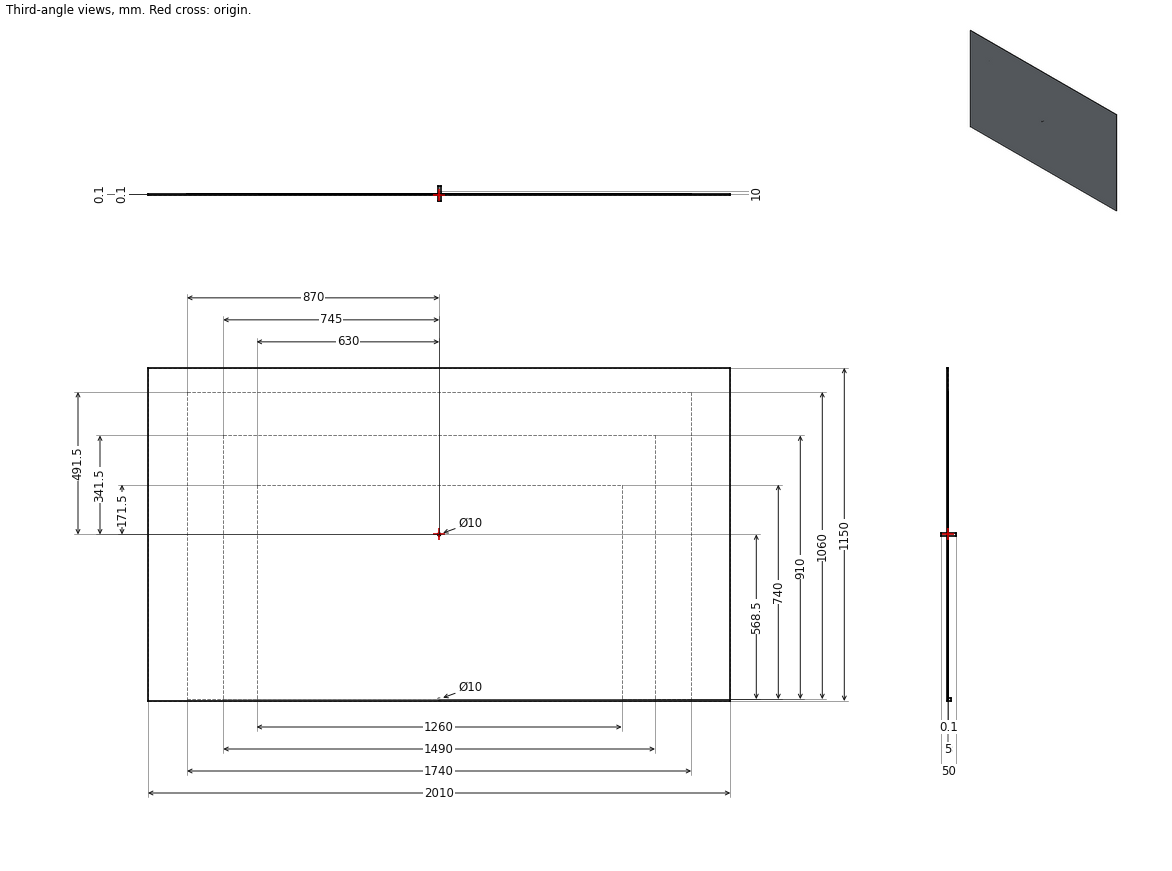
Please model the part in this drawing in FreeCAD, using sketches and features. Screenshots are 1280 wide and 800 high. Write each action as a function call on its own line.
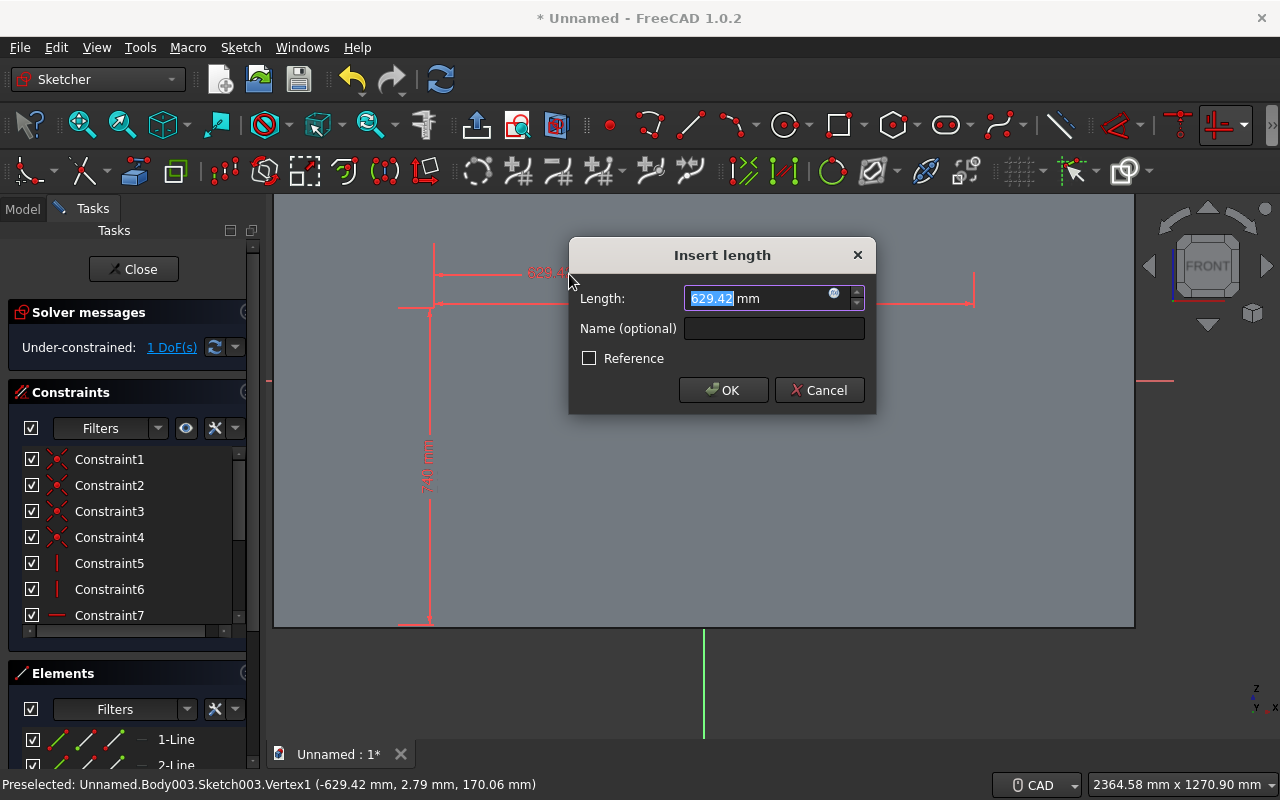
text(630)
key(Return)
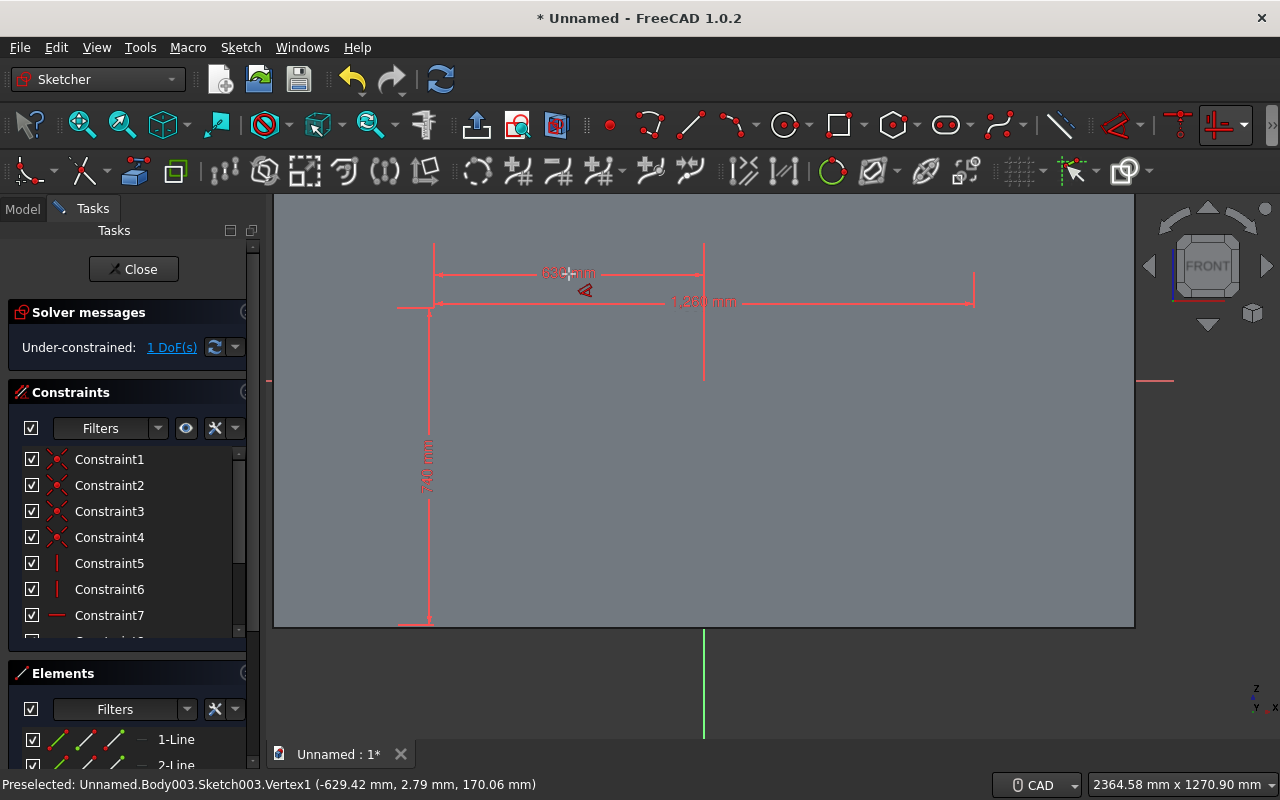
click(434, 308)
click(400, 344)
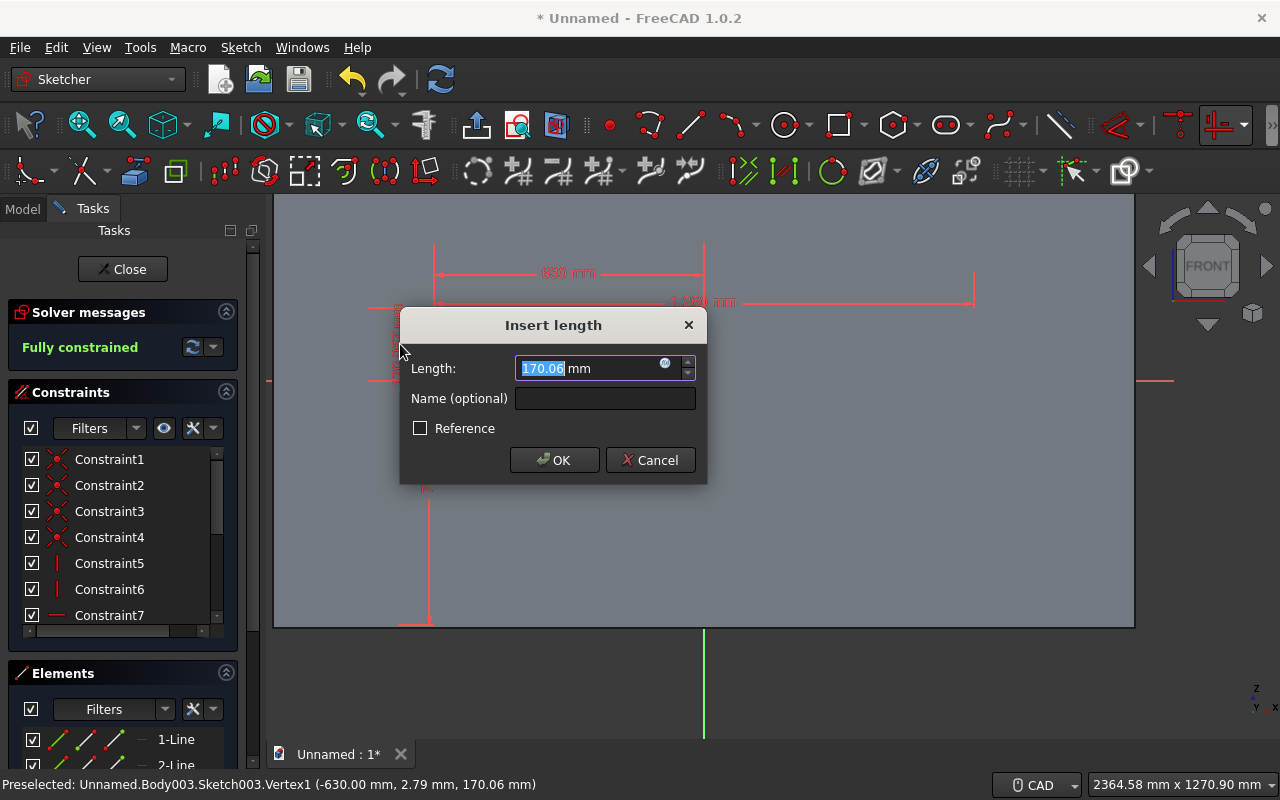
text(171.5)
key(Return)
key(Escape)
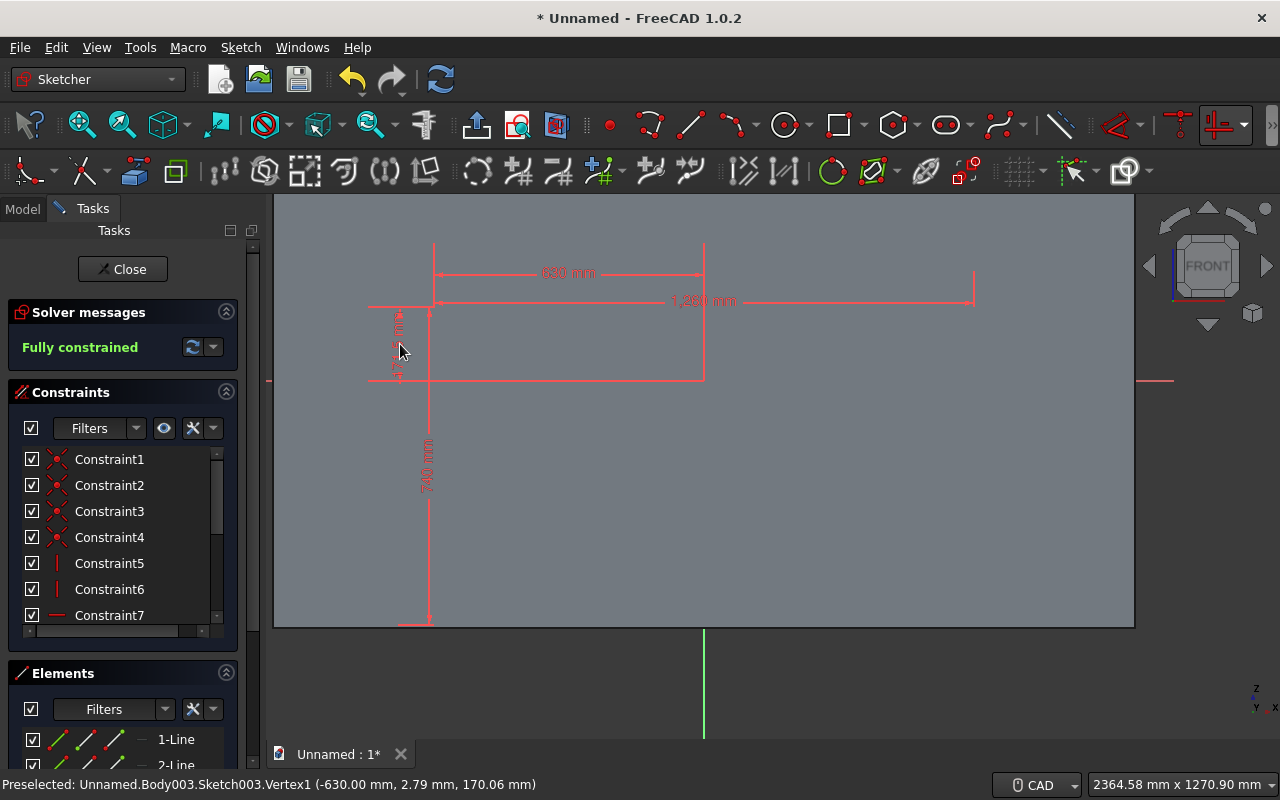
click(123, 269)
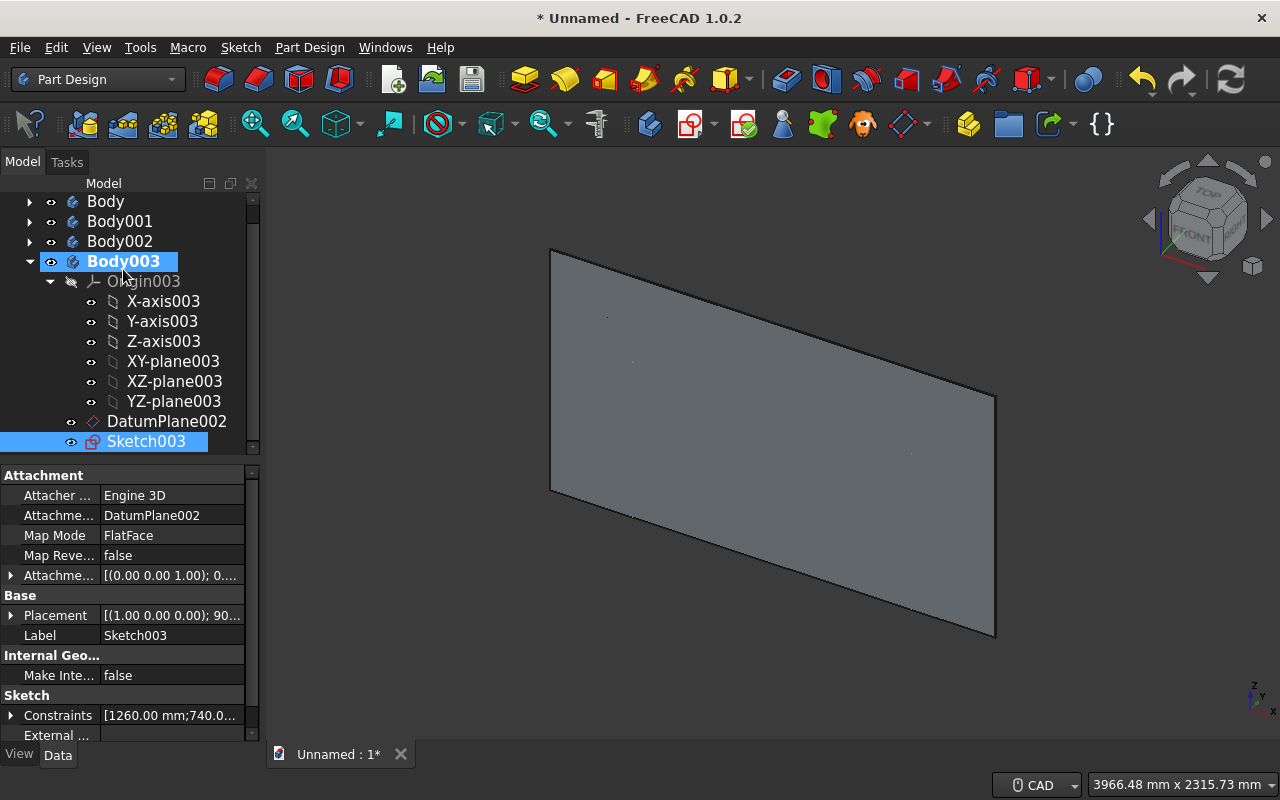
click(526, 80)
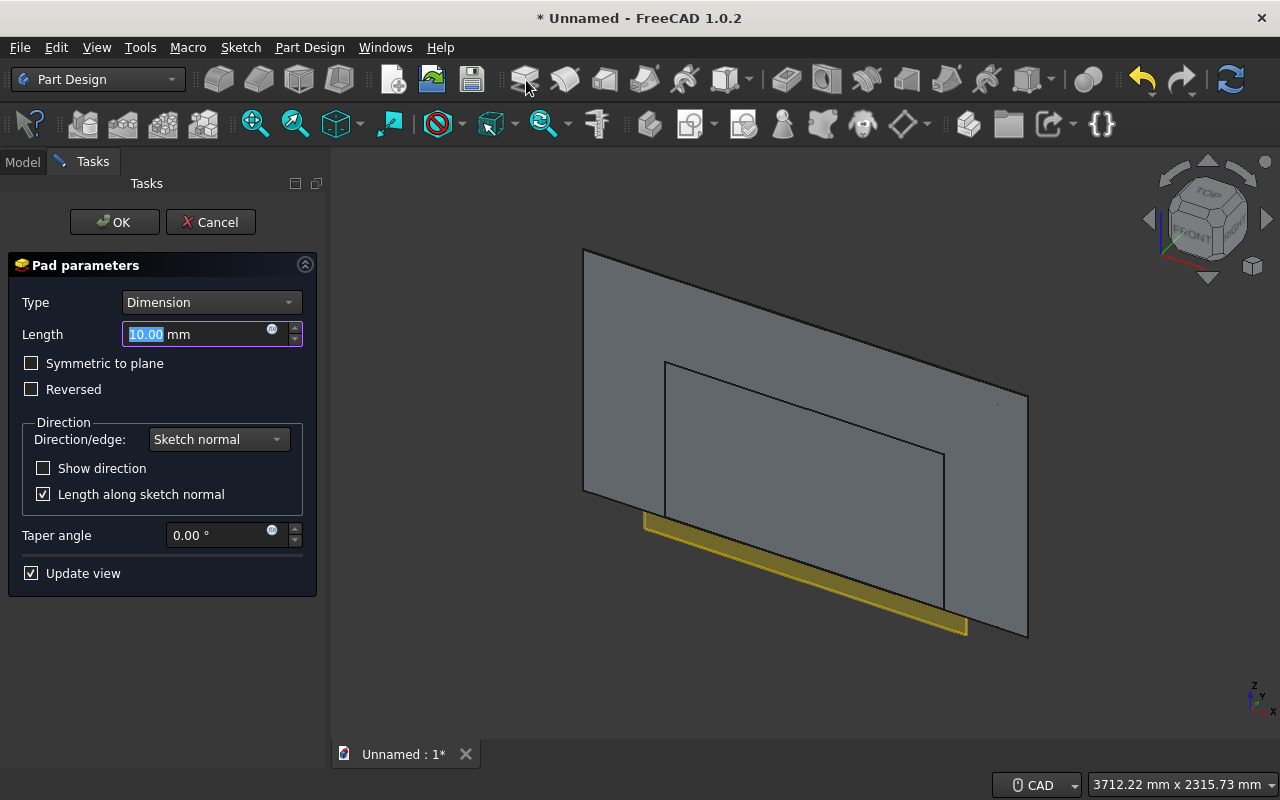
text(0.1)
key(Tab)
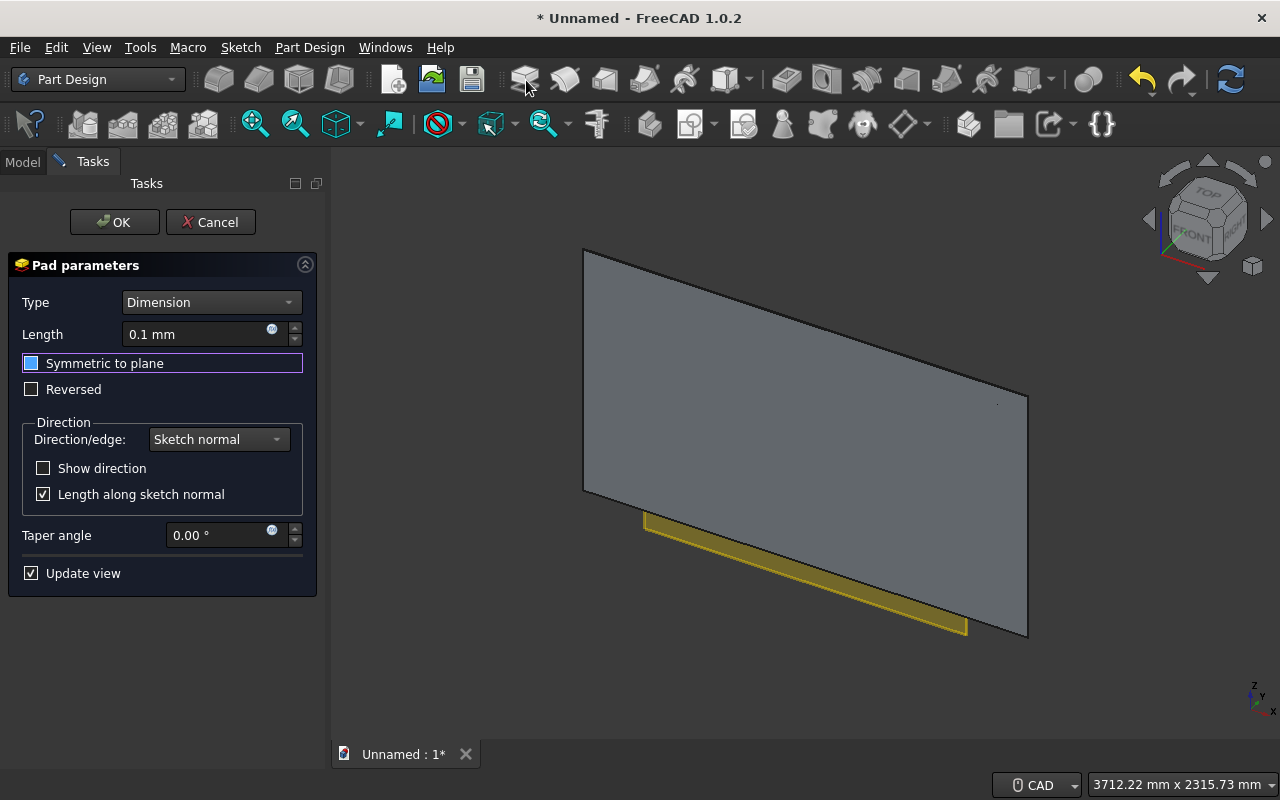
click(30, 389)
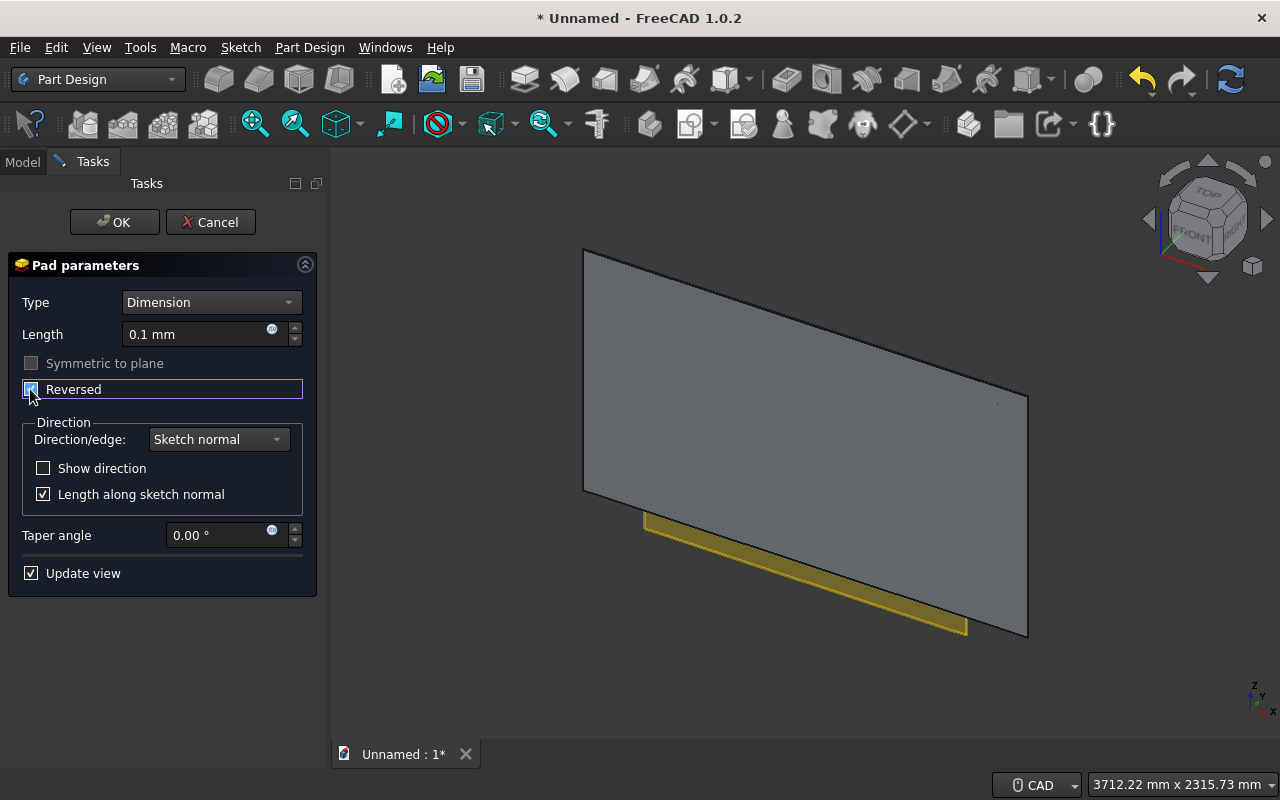
click(115, 222)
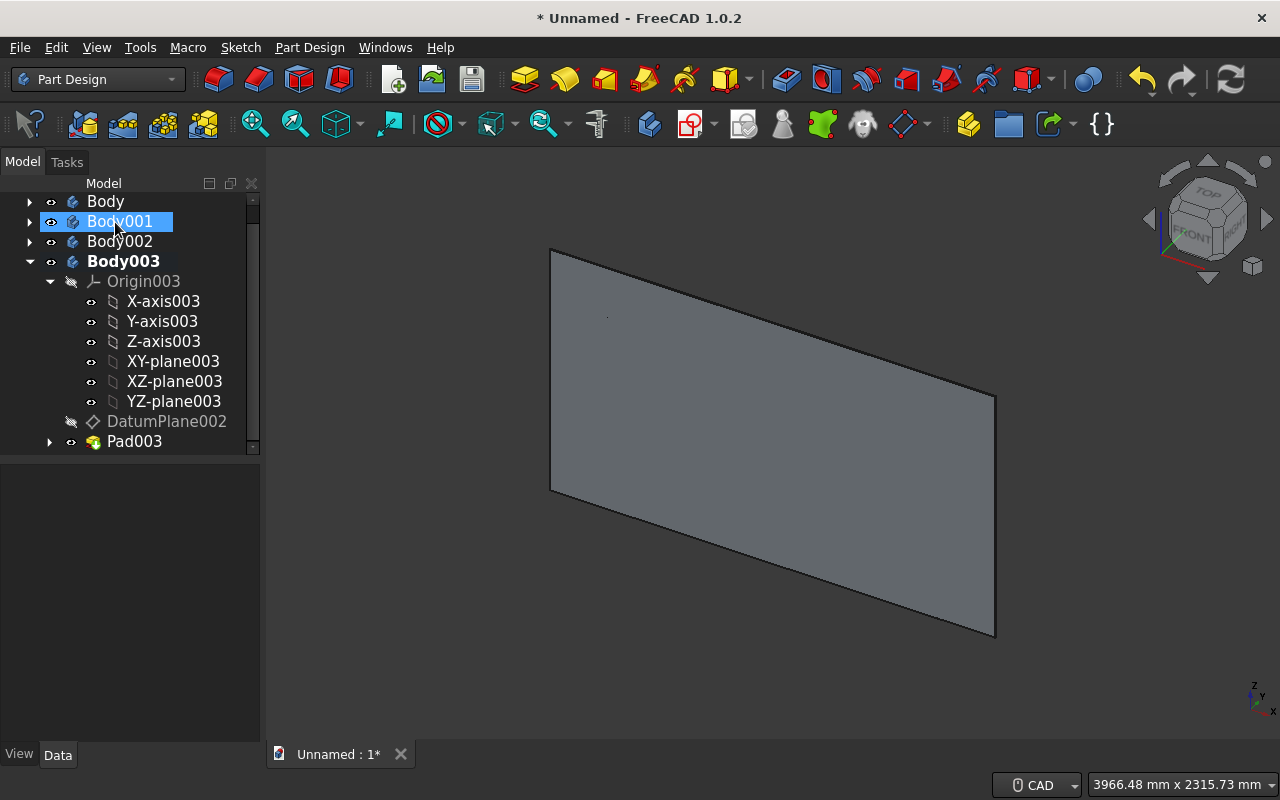
click(256, 124)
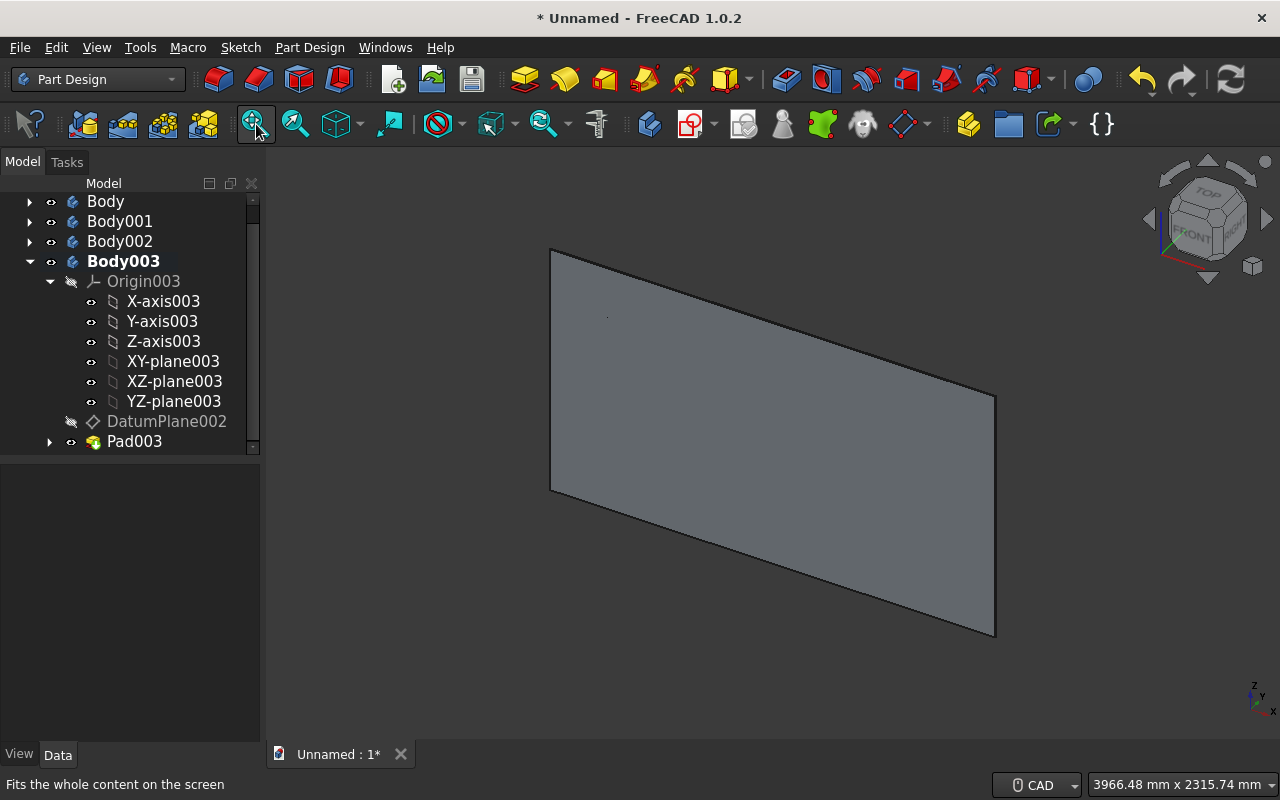
key(4)